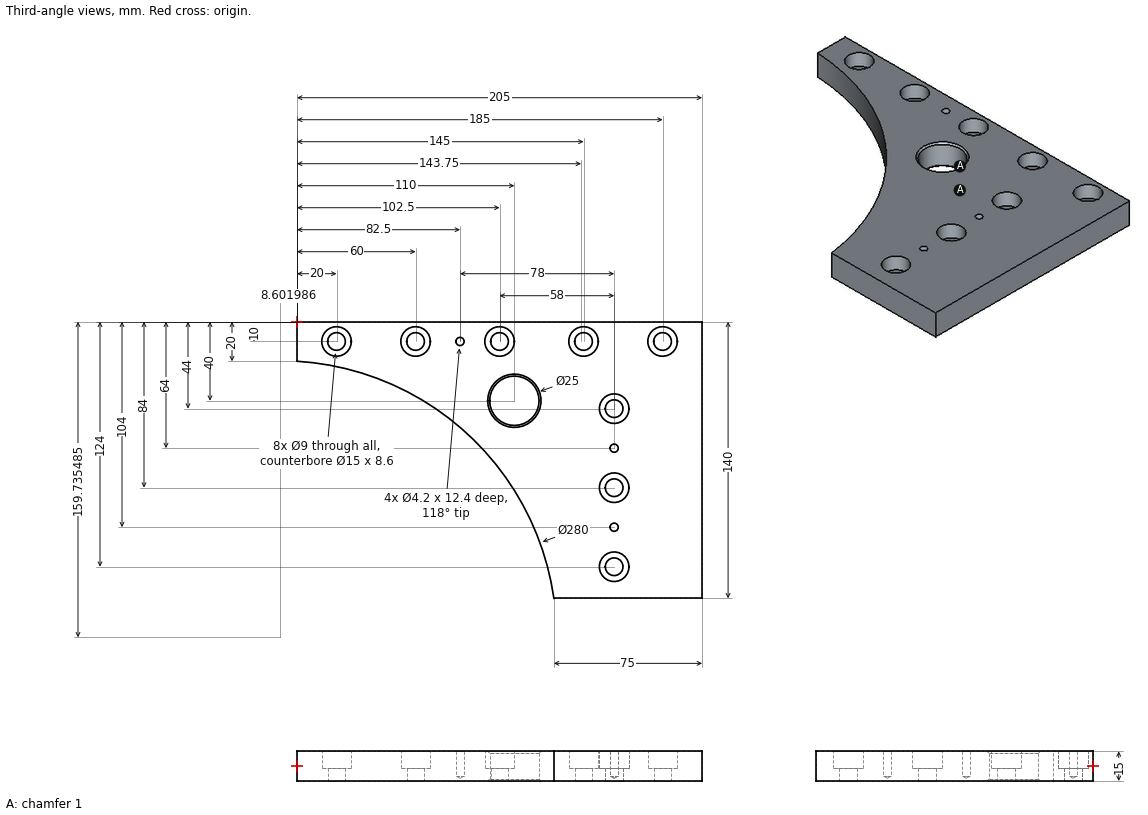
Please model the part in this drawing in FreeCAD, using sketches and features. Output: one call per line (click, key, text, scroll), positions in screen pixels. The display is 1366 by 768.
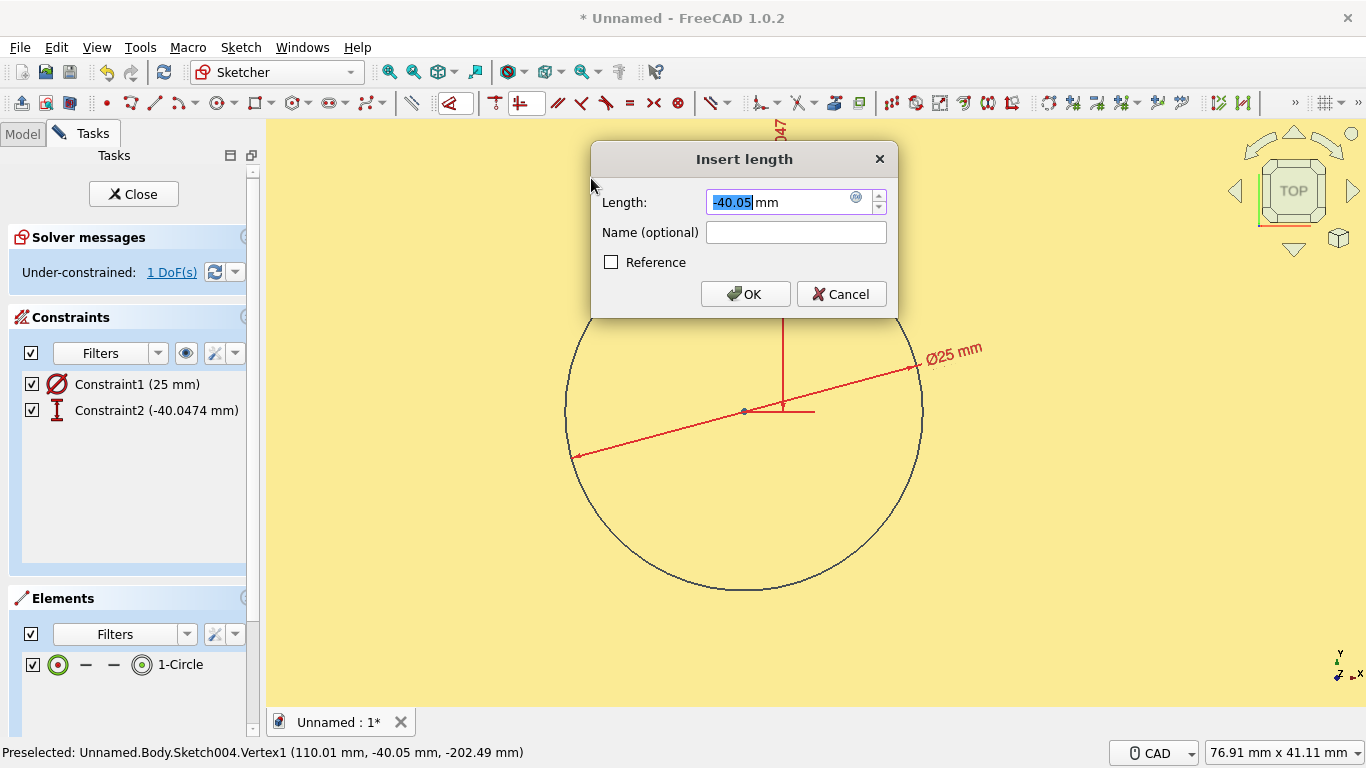
text(-40)
key(Return)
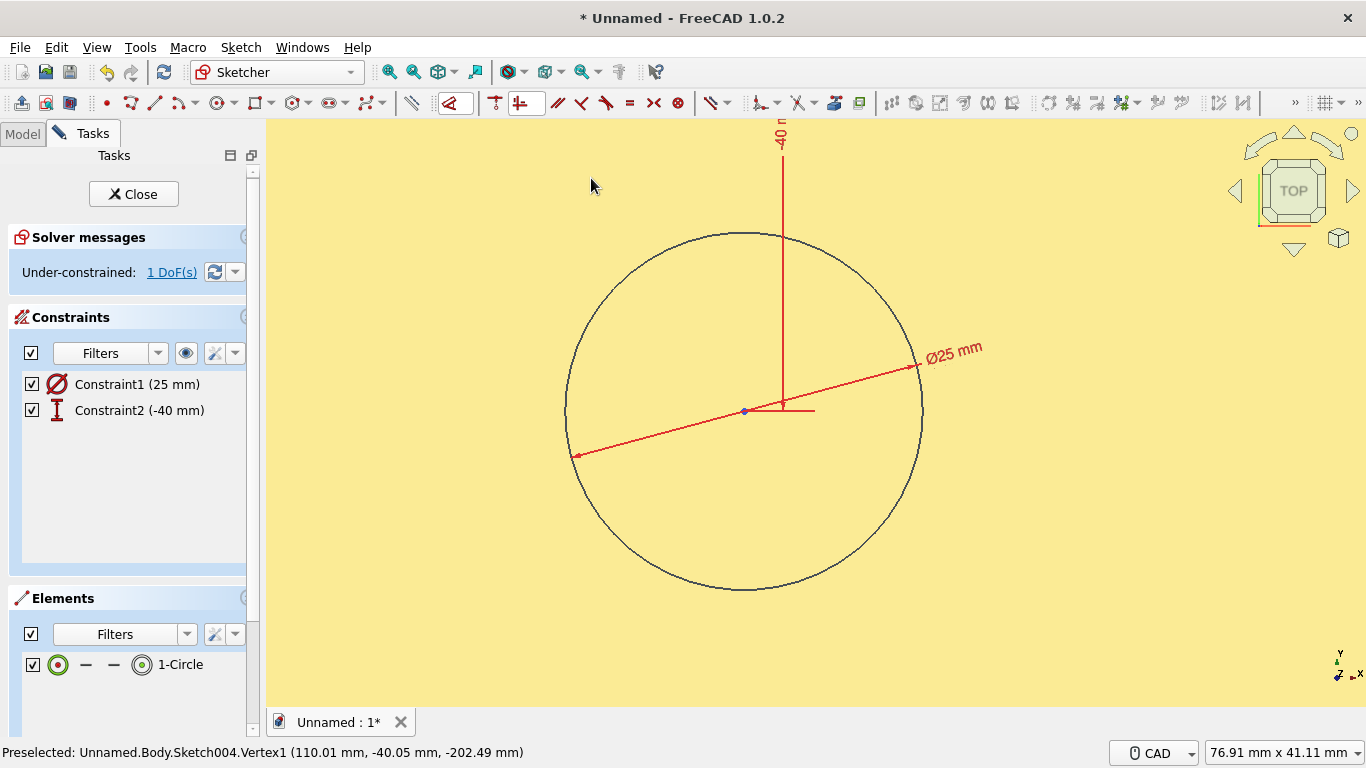
click(744, 411)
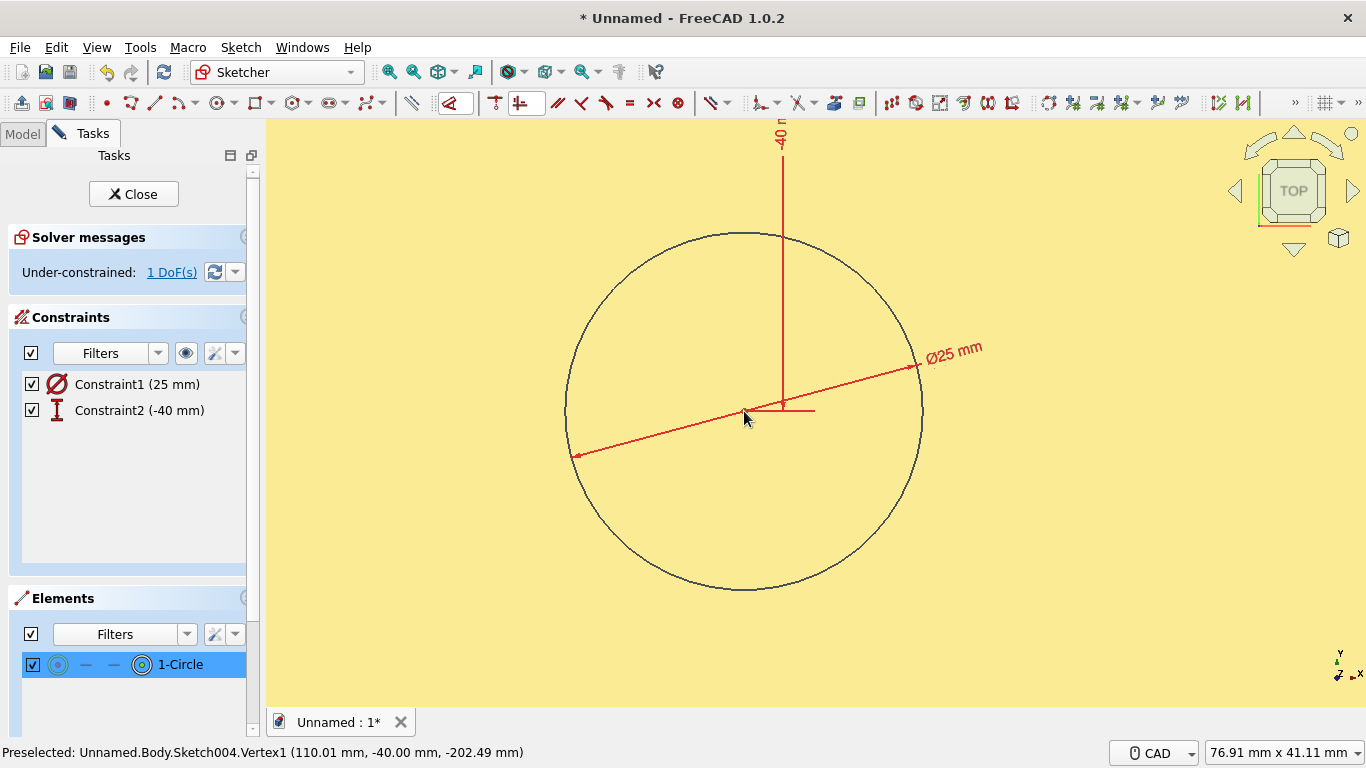
click(468, 104)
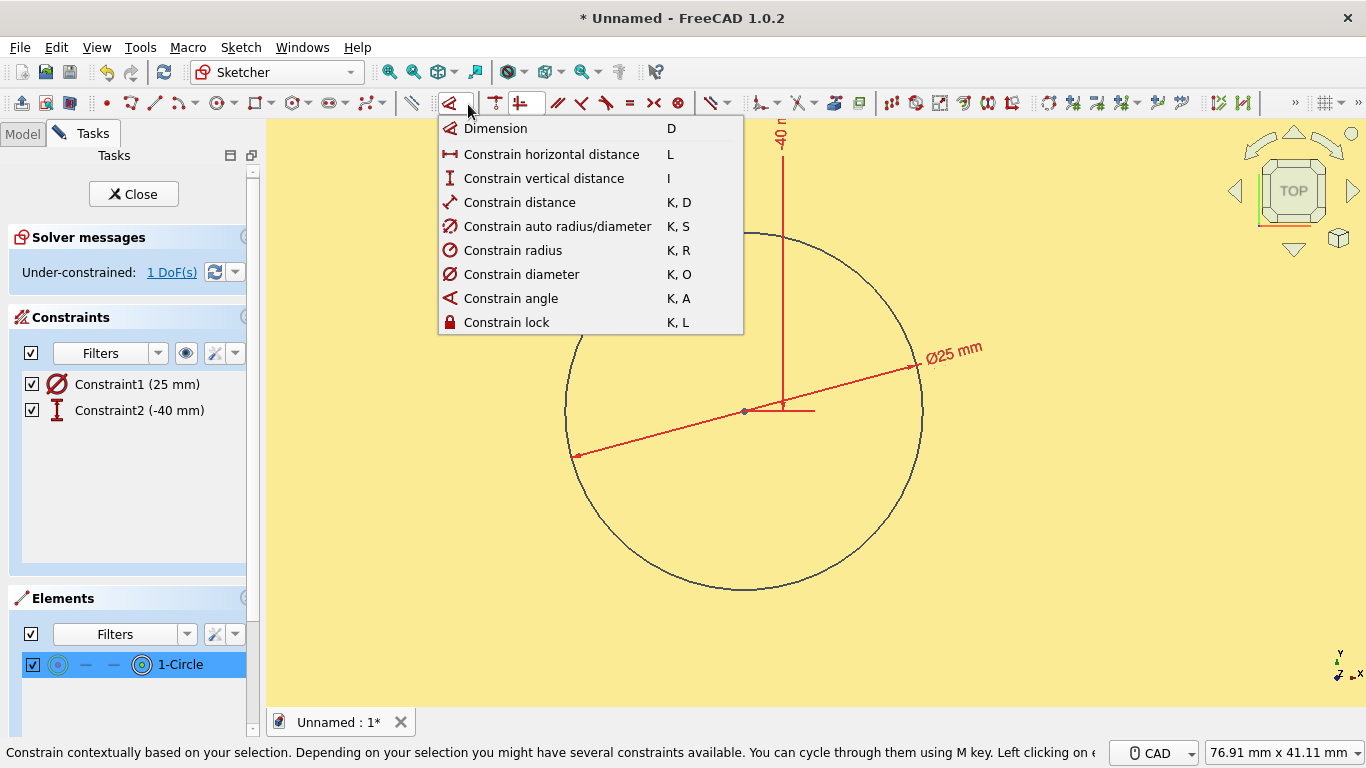
click(591, 154)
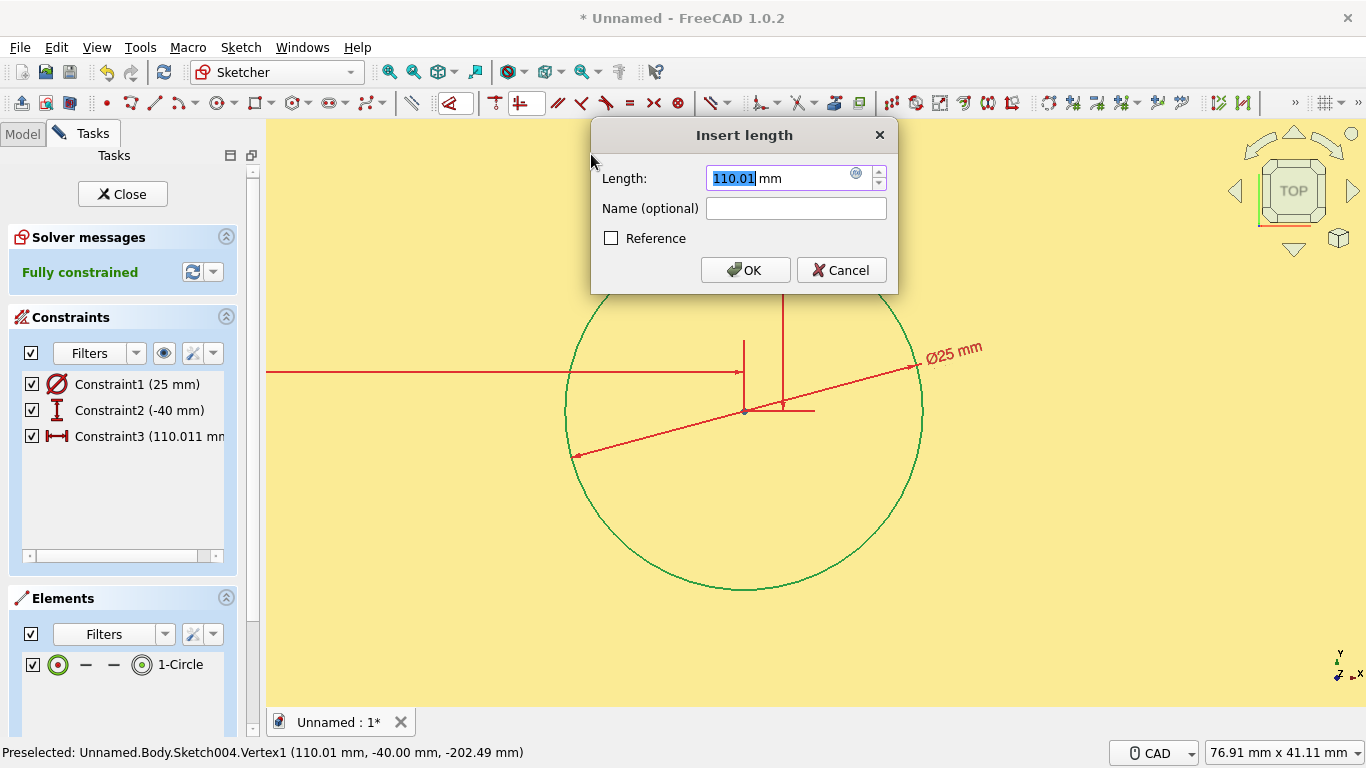
text(110)
key(Return)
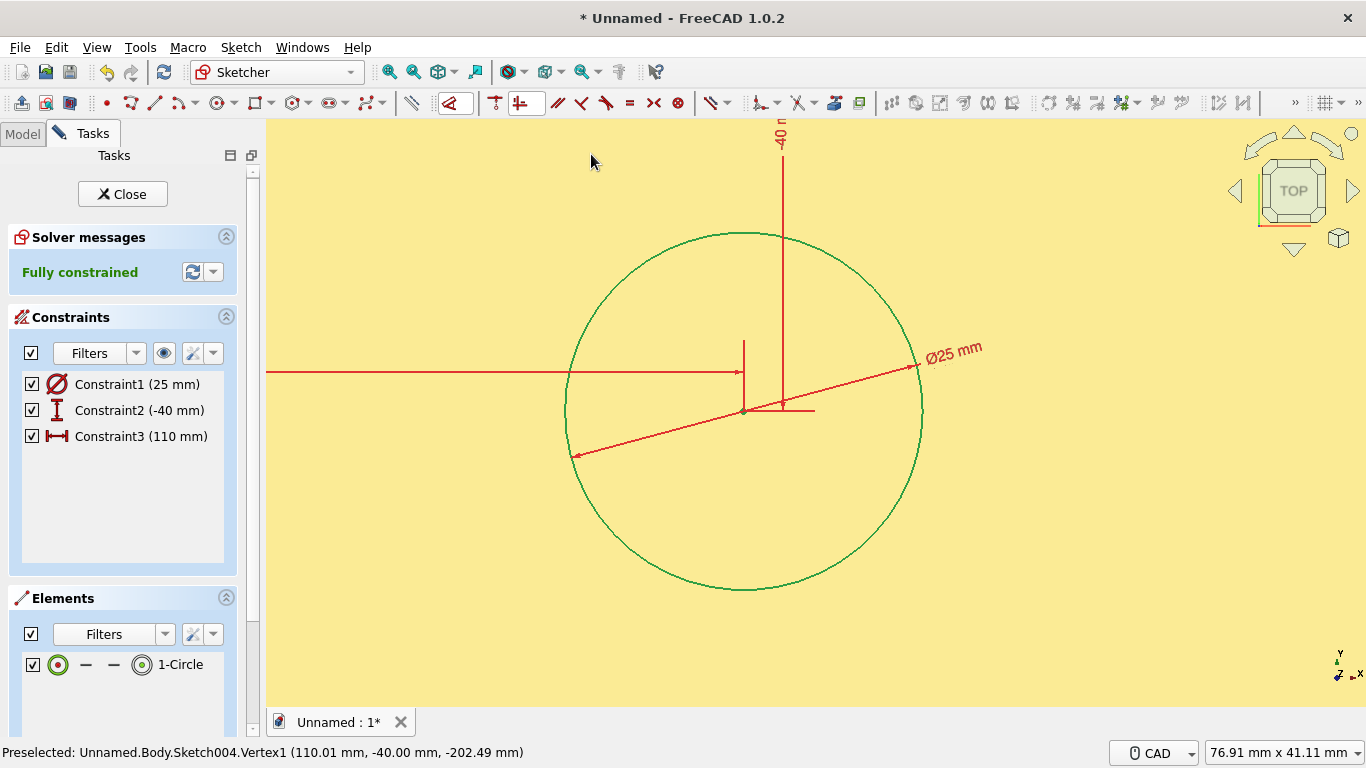
click(123, 194)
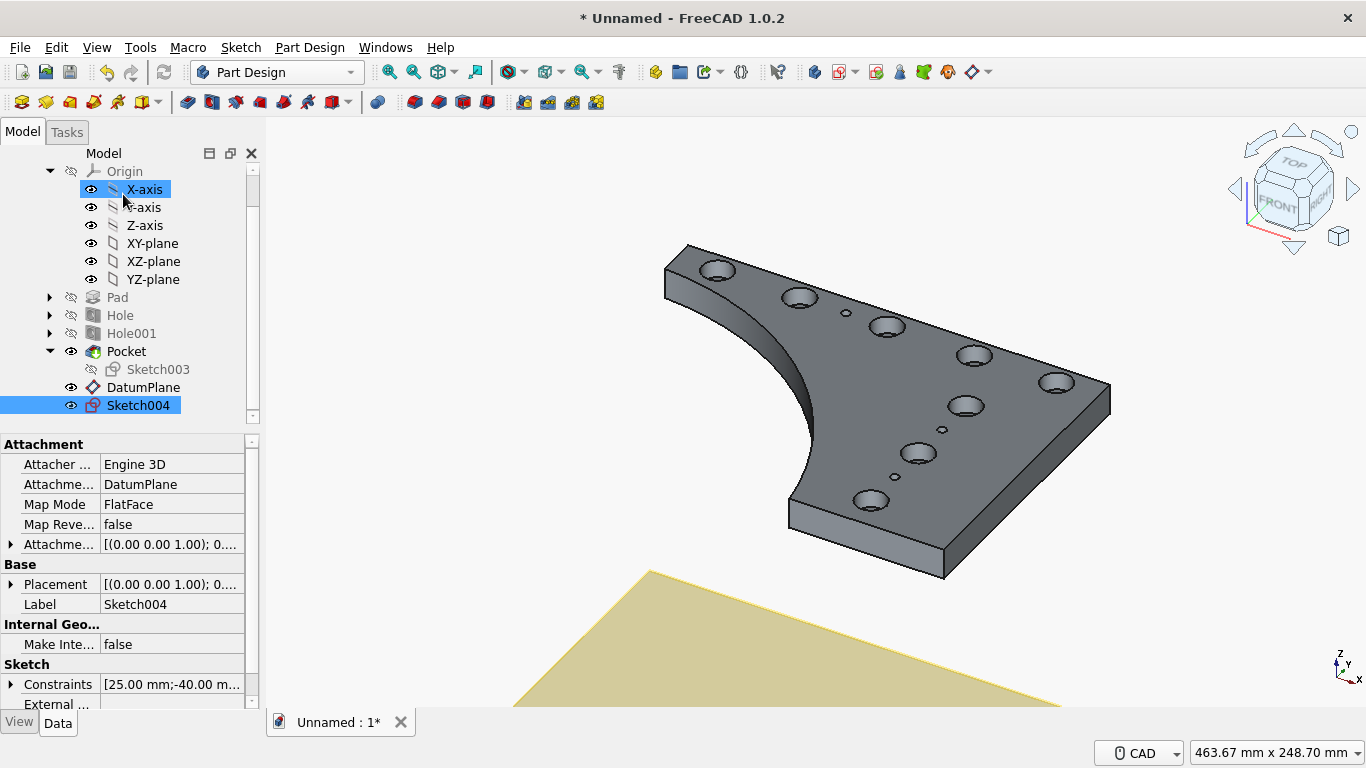
click(188, 102)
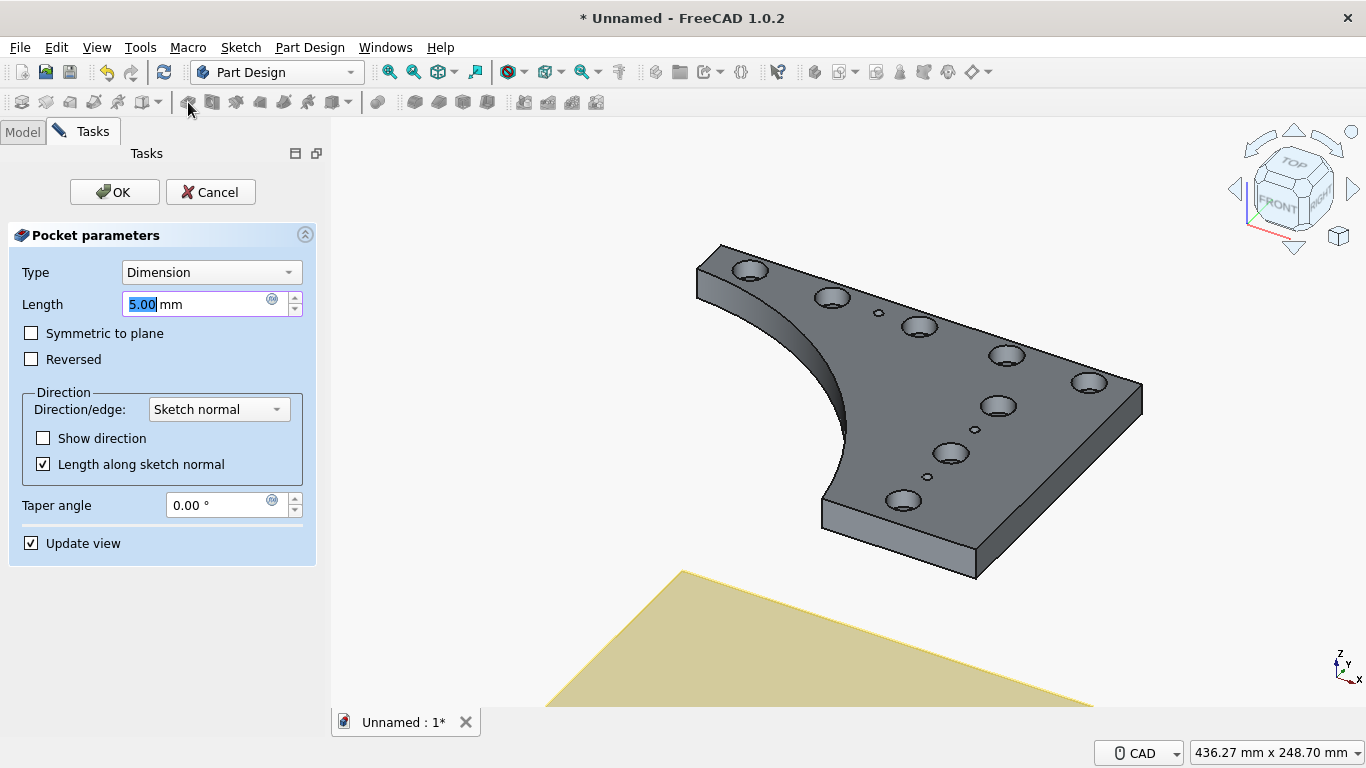
click(212, 272)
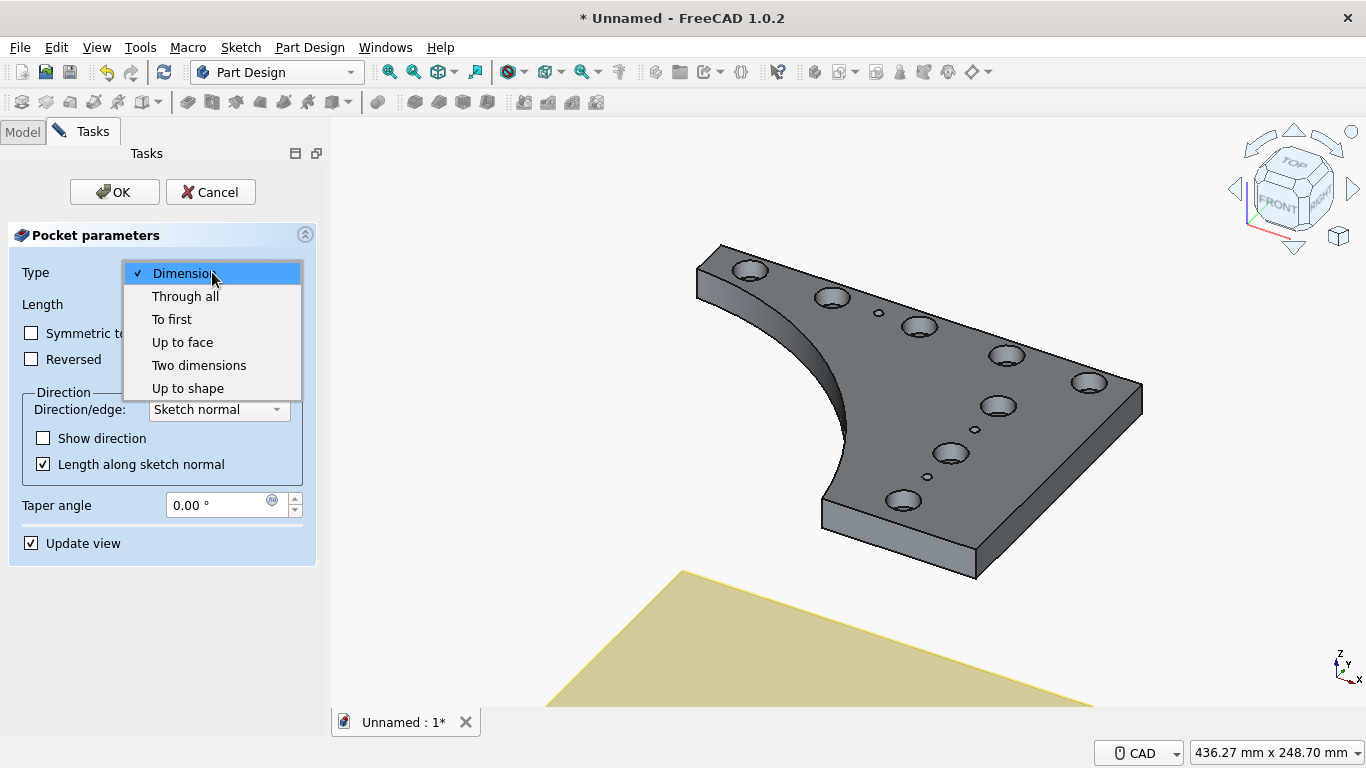
click(212, 296)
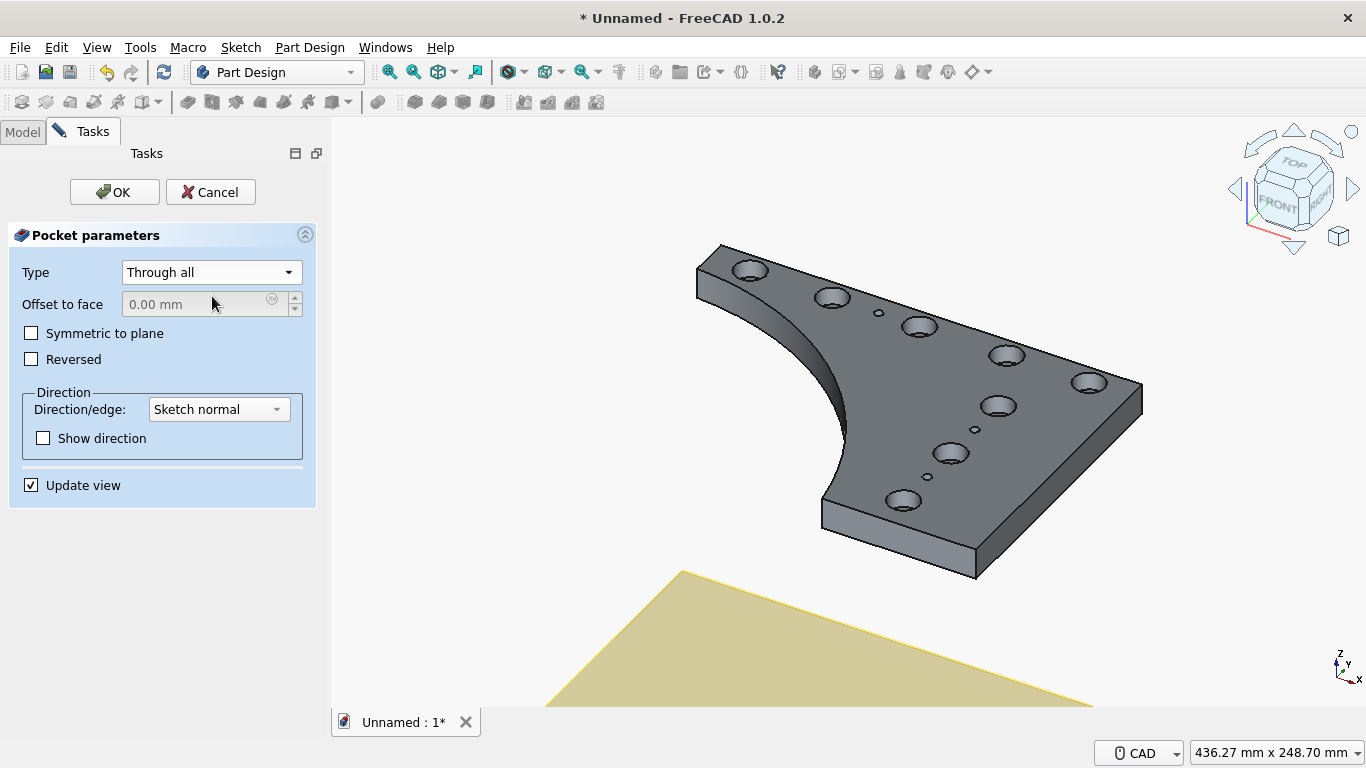
click(30, 359)